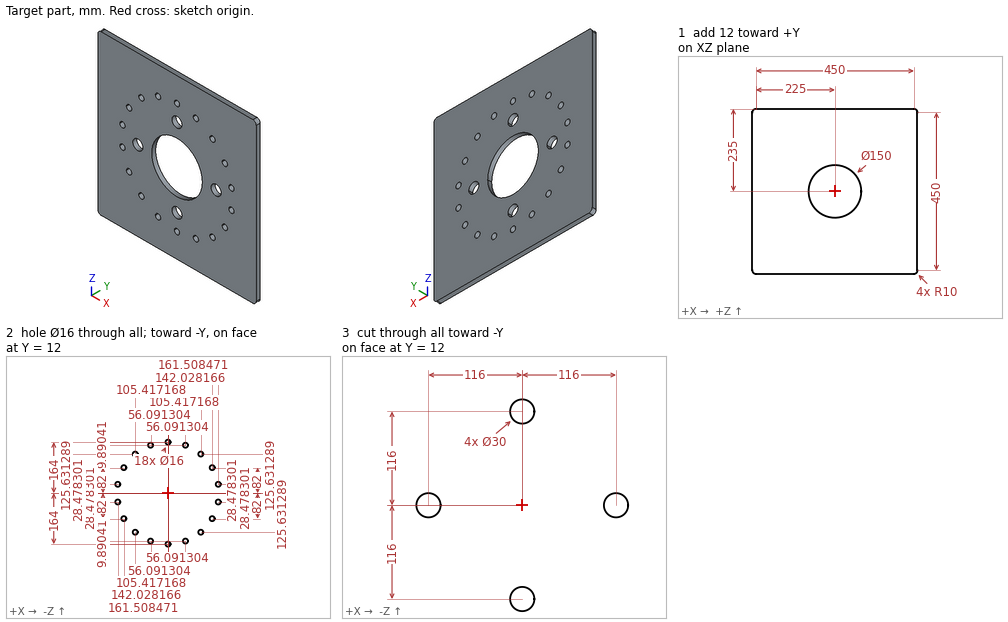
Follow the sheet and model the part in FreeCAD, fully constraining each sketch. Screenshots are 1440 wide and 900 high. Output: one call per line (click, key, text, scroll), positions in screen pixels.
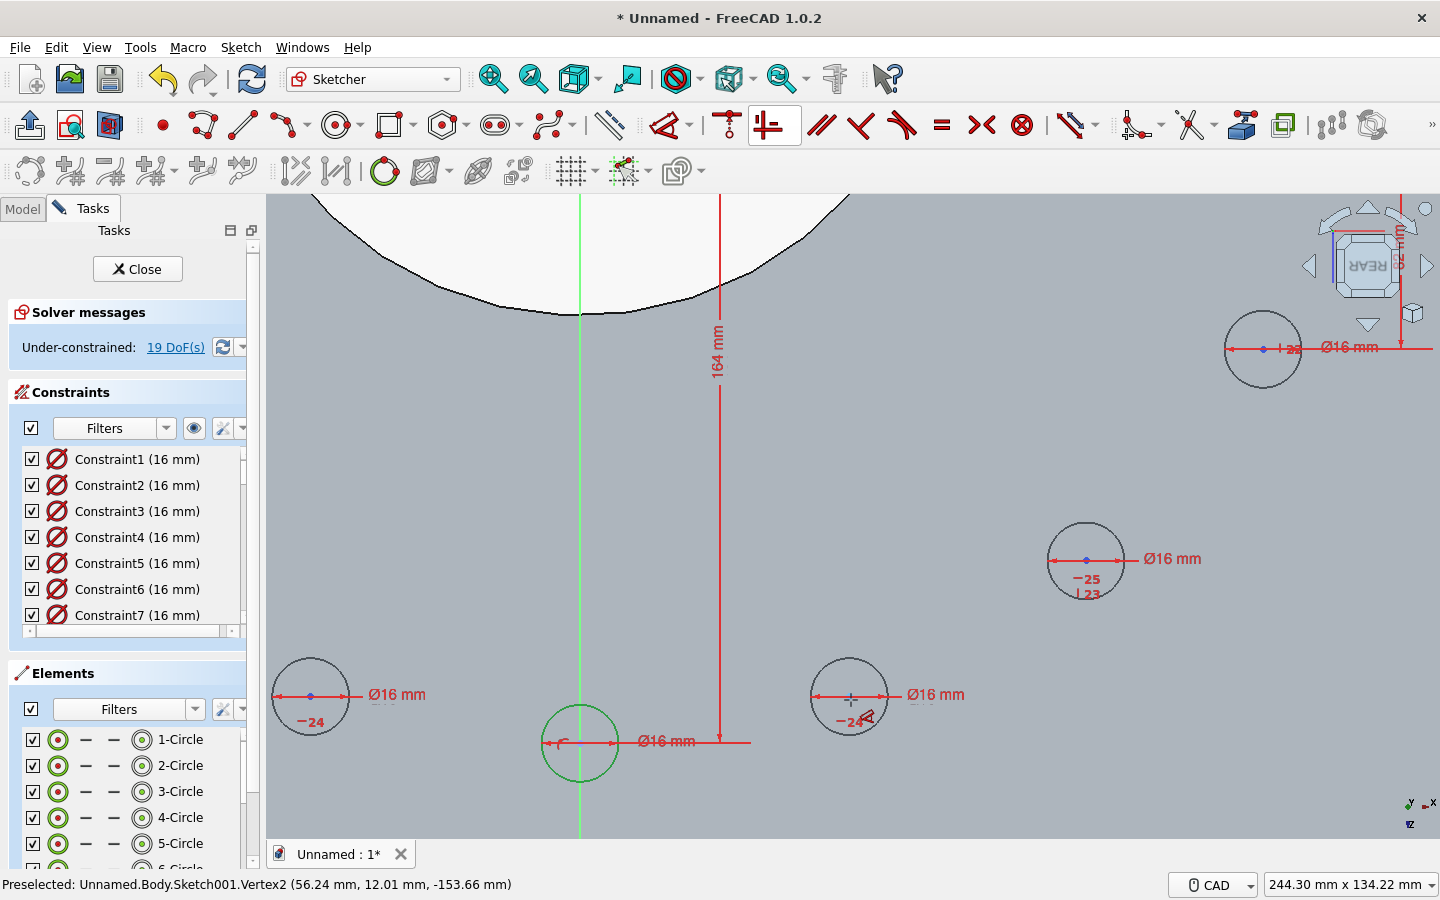
click(849, 697)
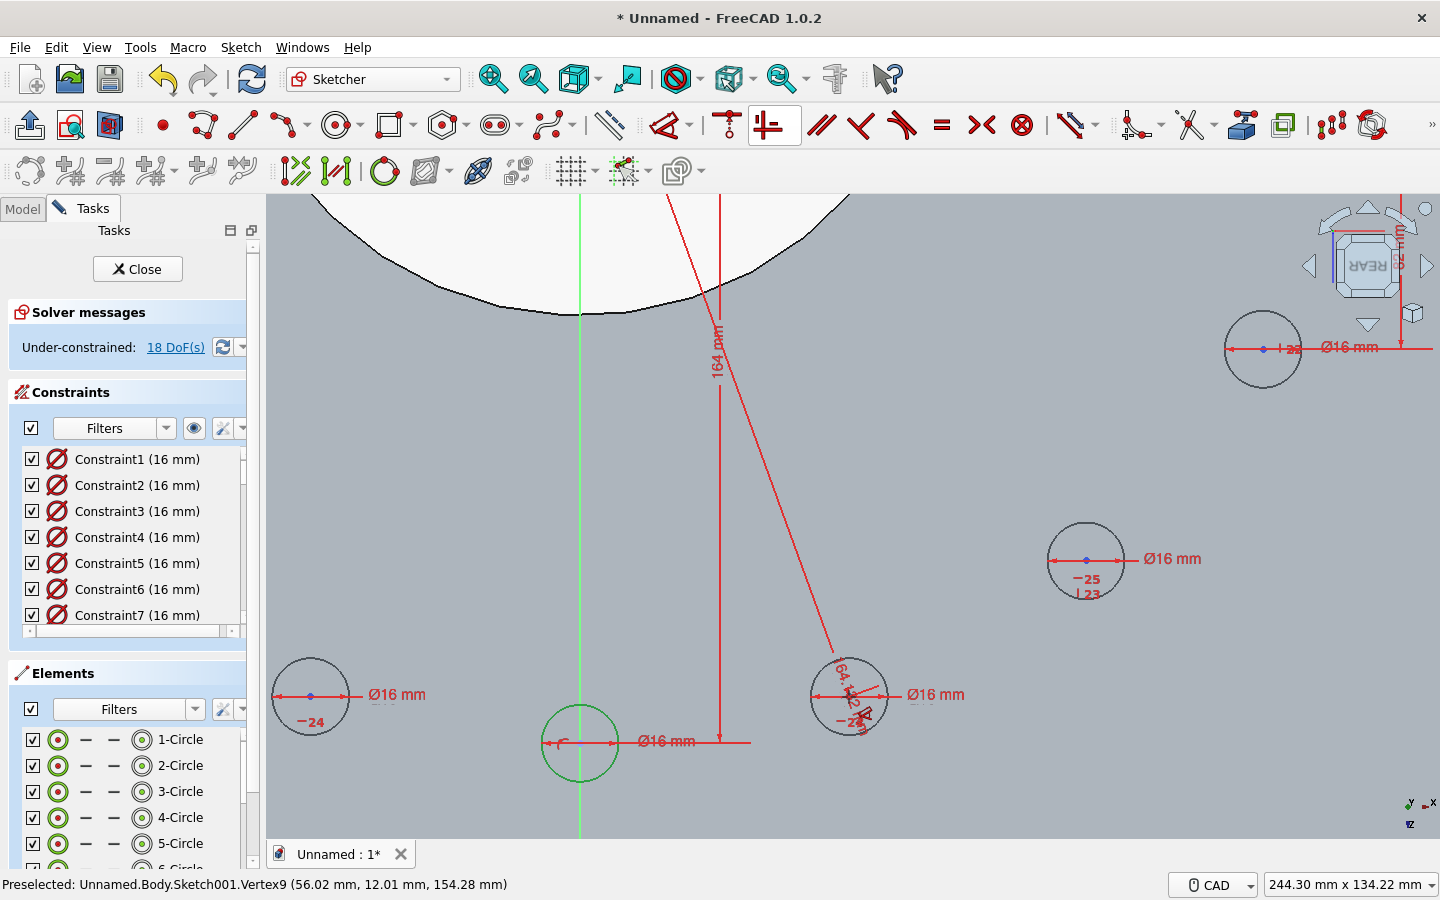
click(580, 743)
click(883, 736)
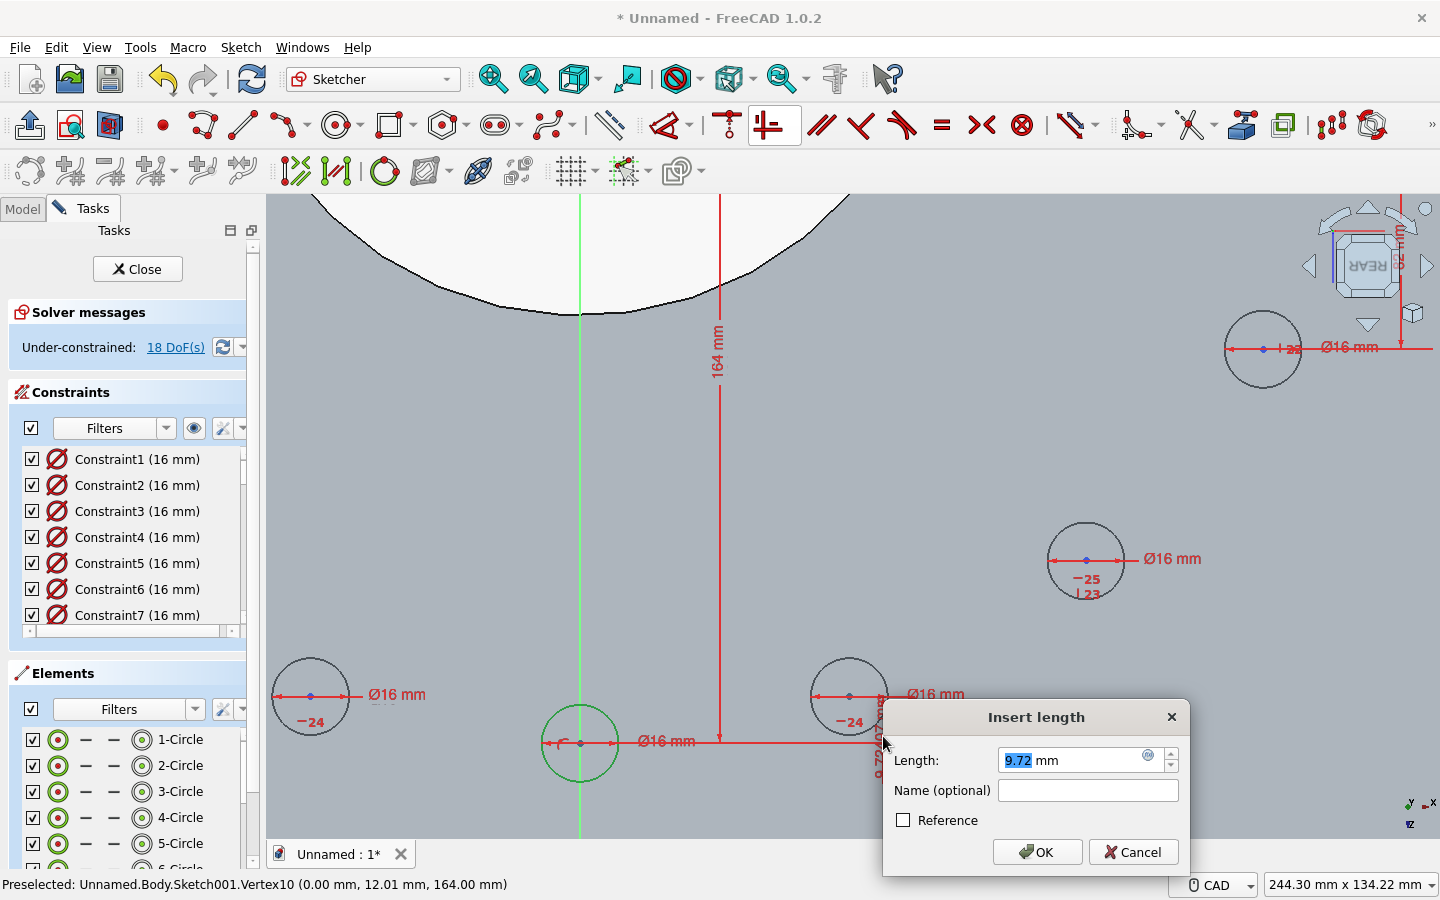
text(9.89041)
key(Return)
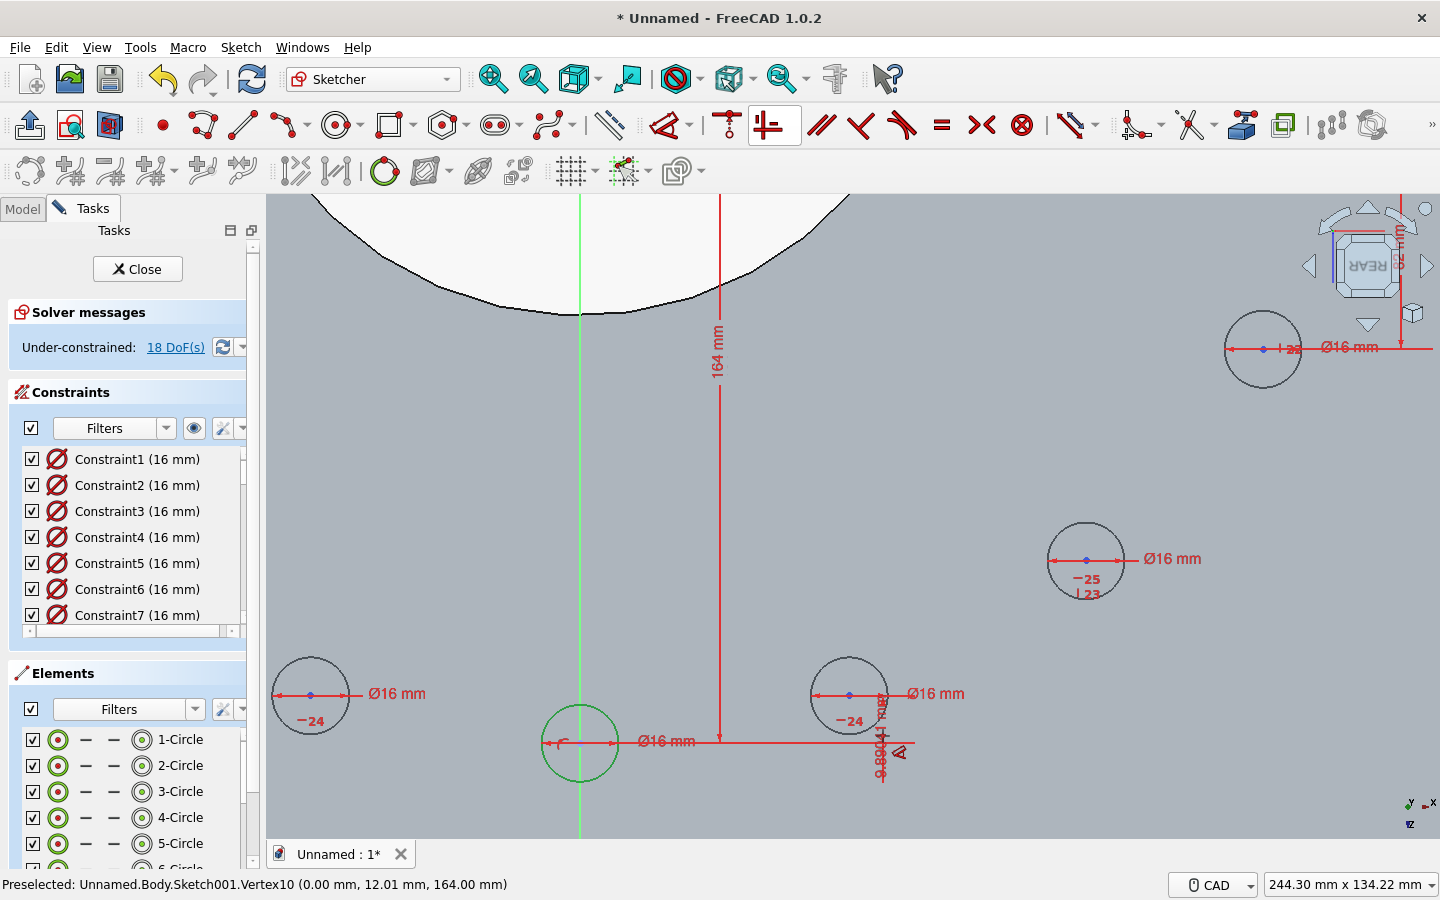
scroll(851, 700, down, 7)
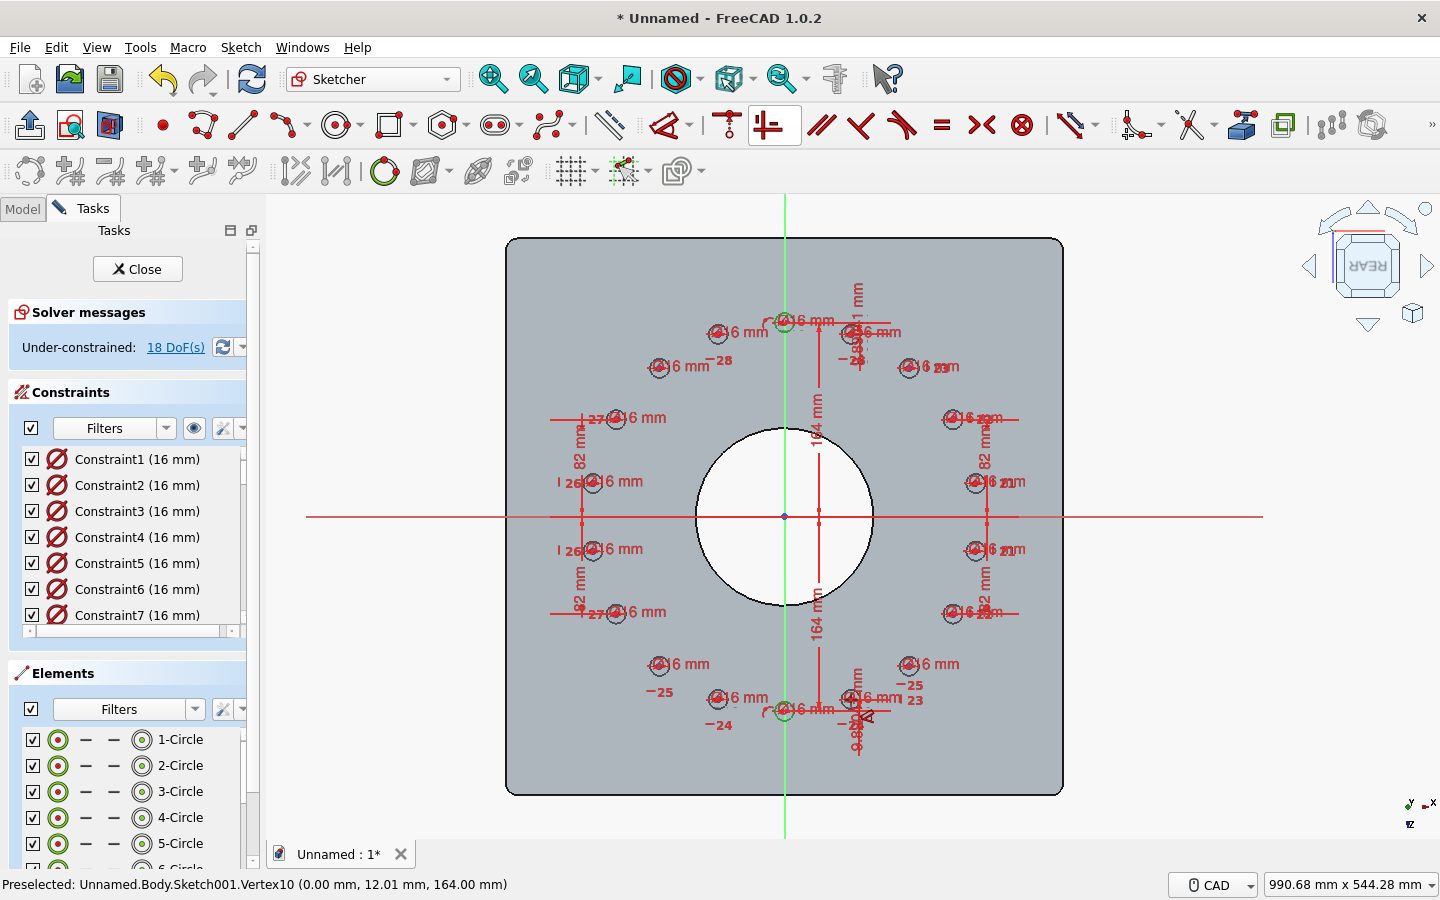
click(851, 334)
click(818, 300)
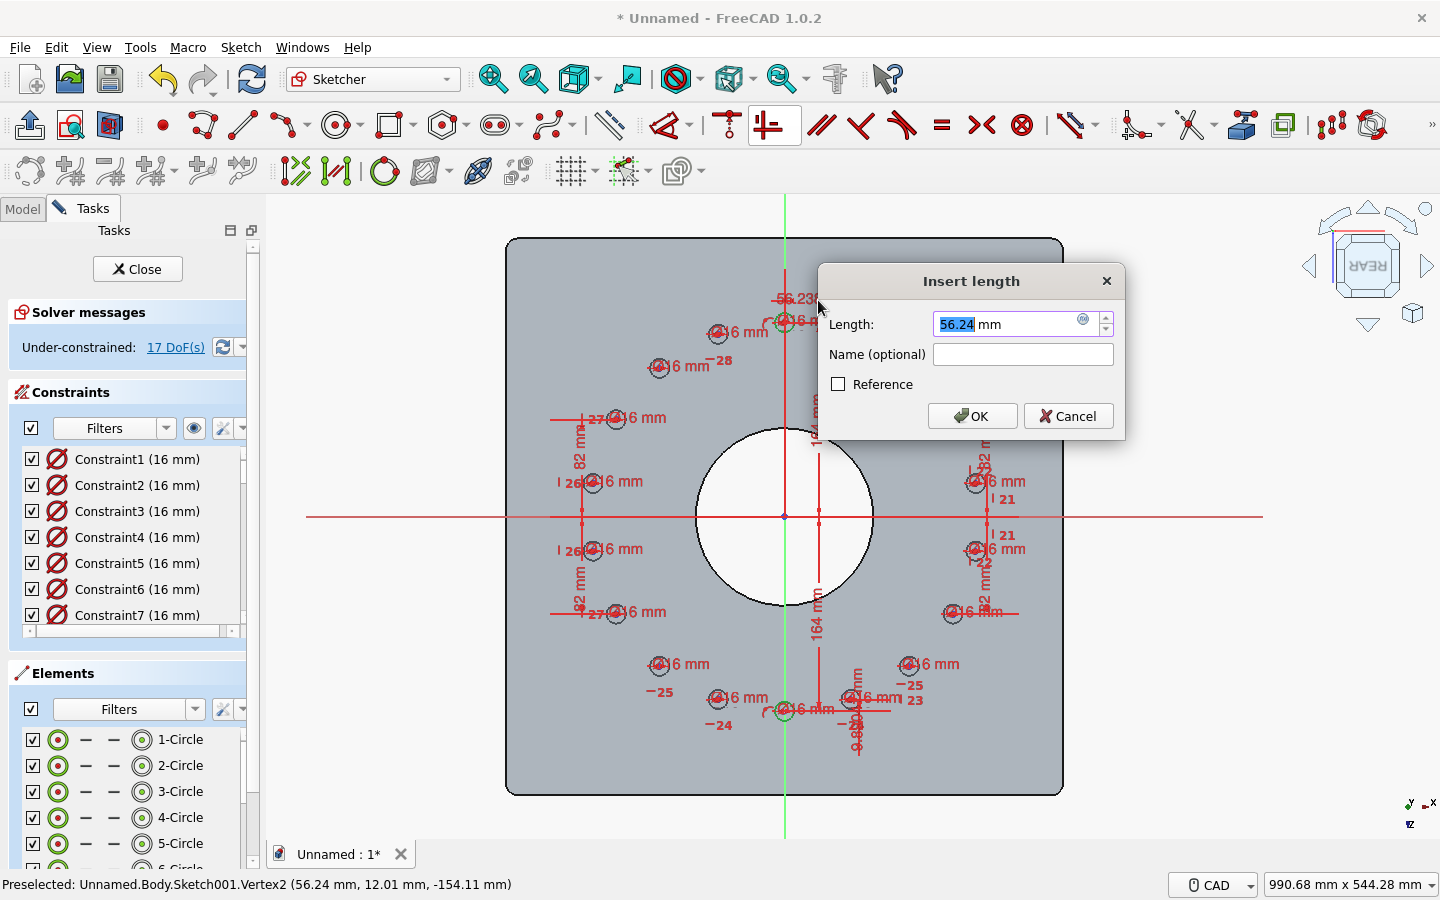
text(56.091304)
key(Return)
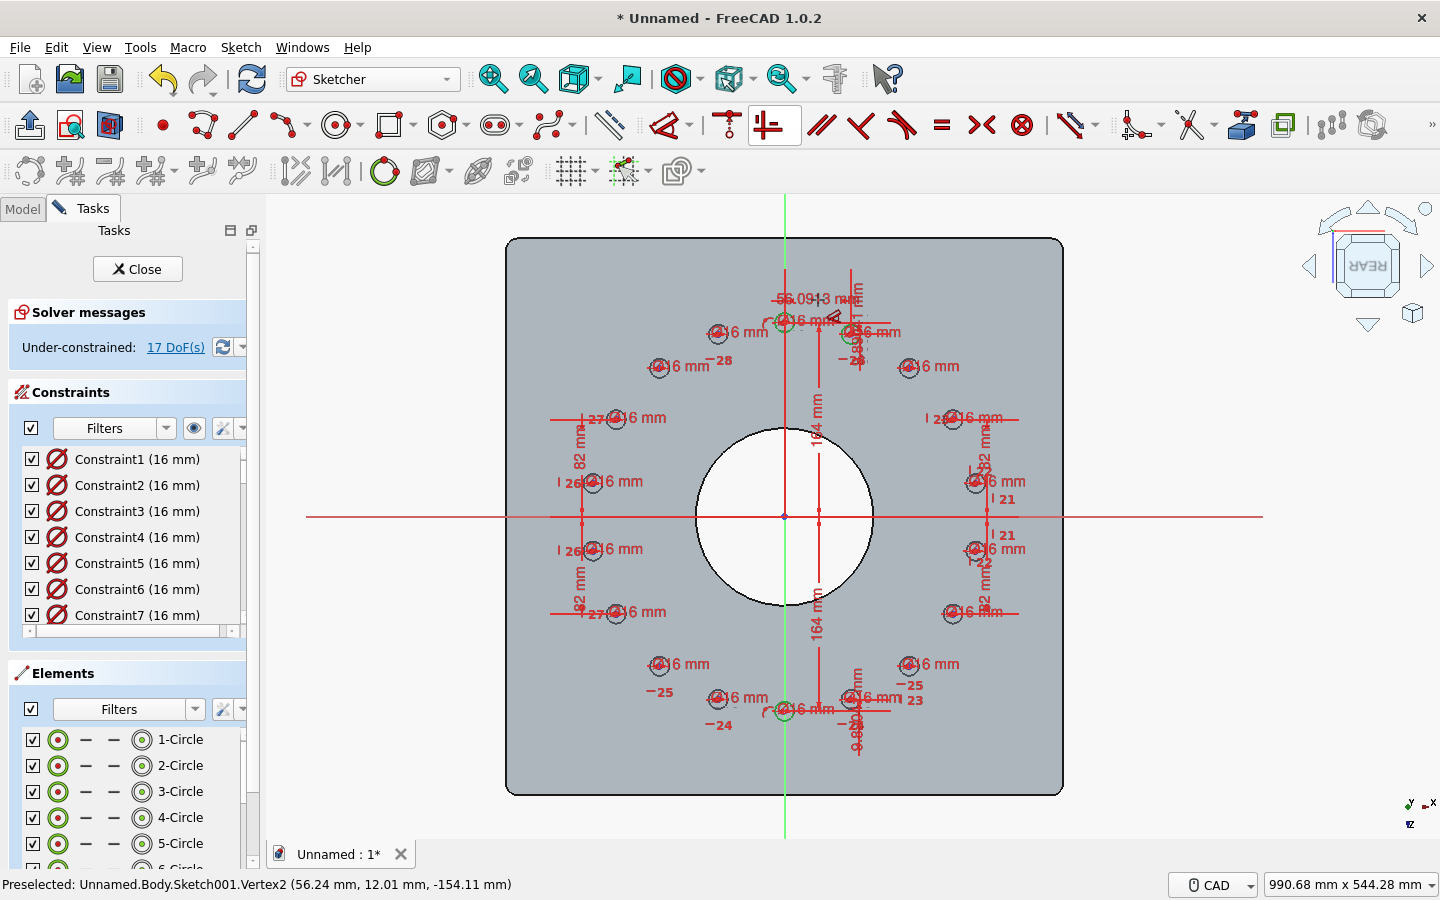
click(976, 483)
click(1010, 500)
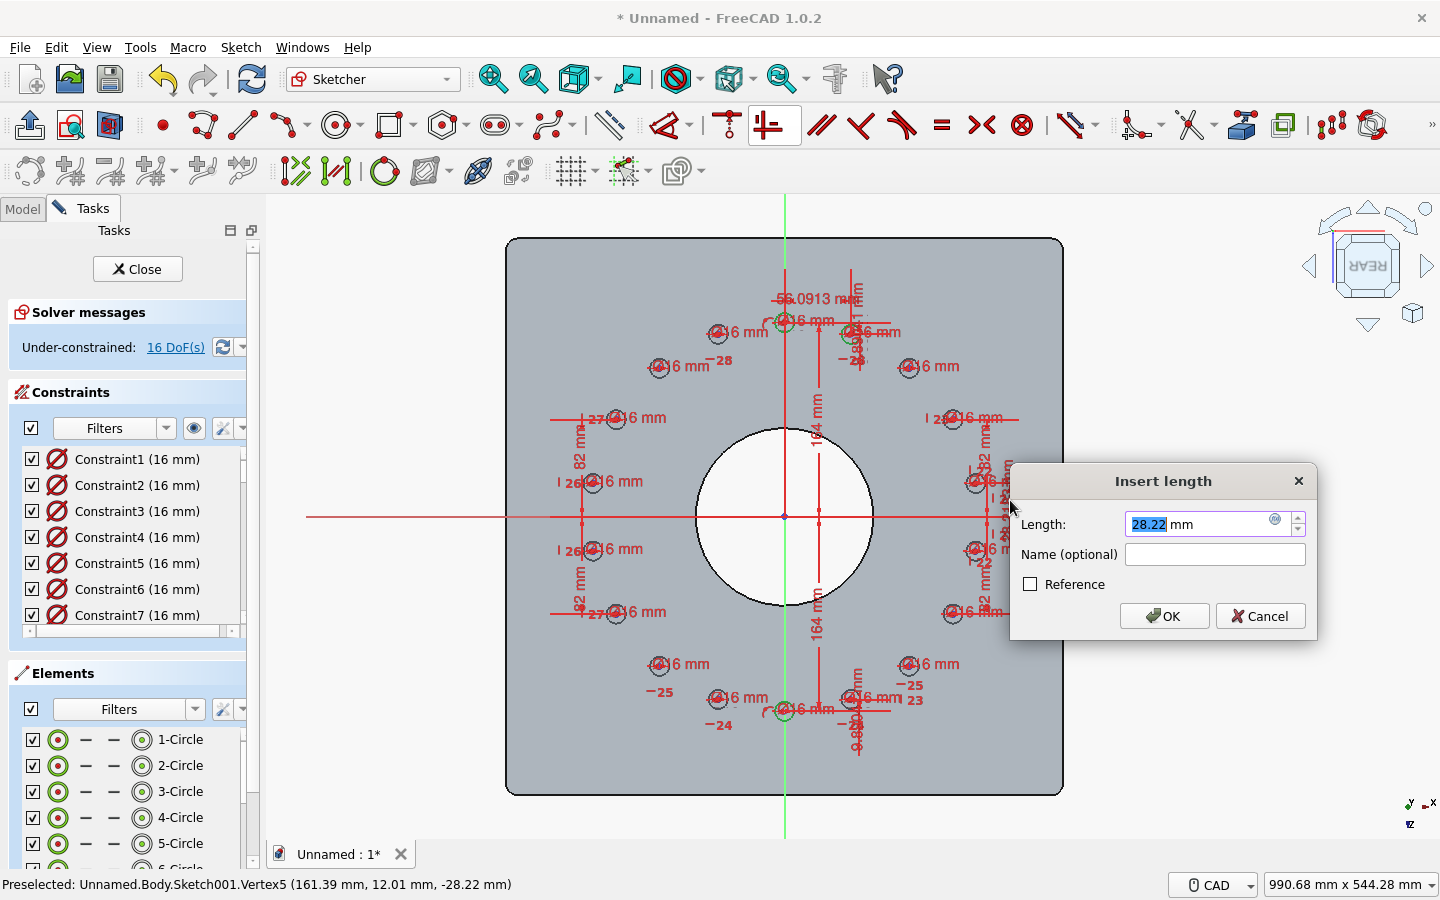
text(28.478301)
key(Return)